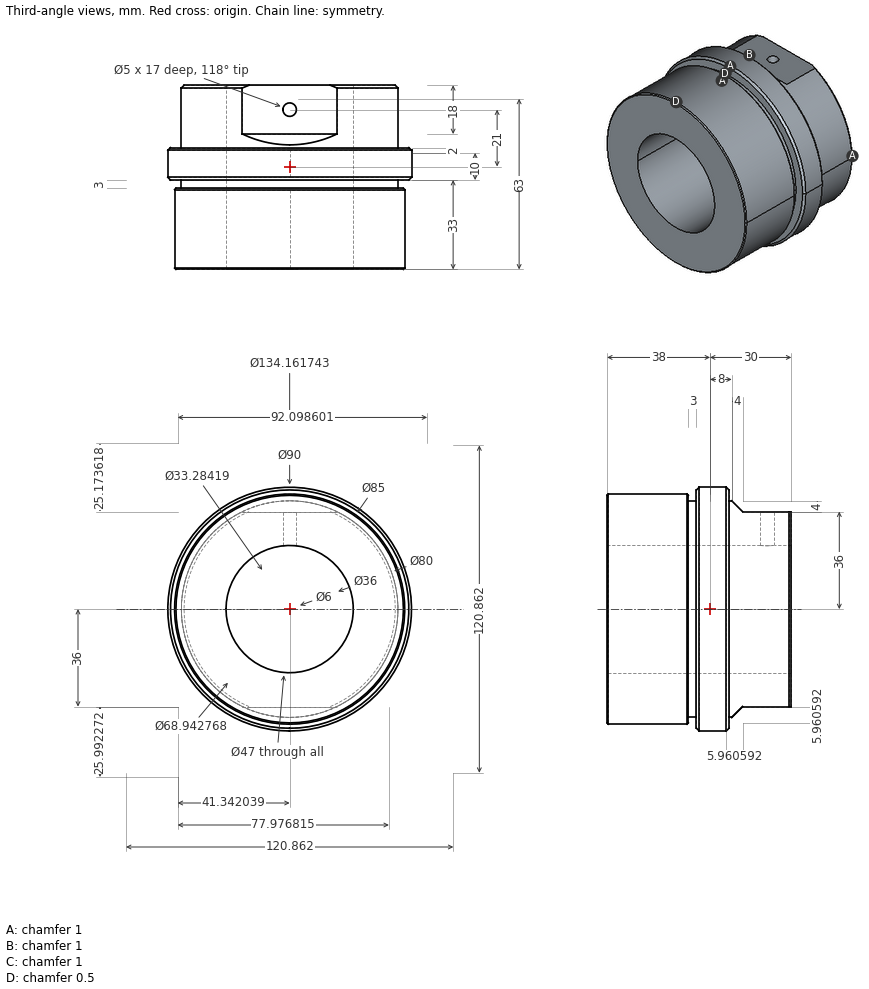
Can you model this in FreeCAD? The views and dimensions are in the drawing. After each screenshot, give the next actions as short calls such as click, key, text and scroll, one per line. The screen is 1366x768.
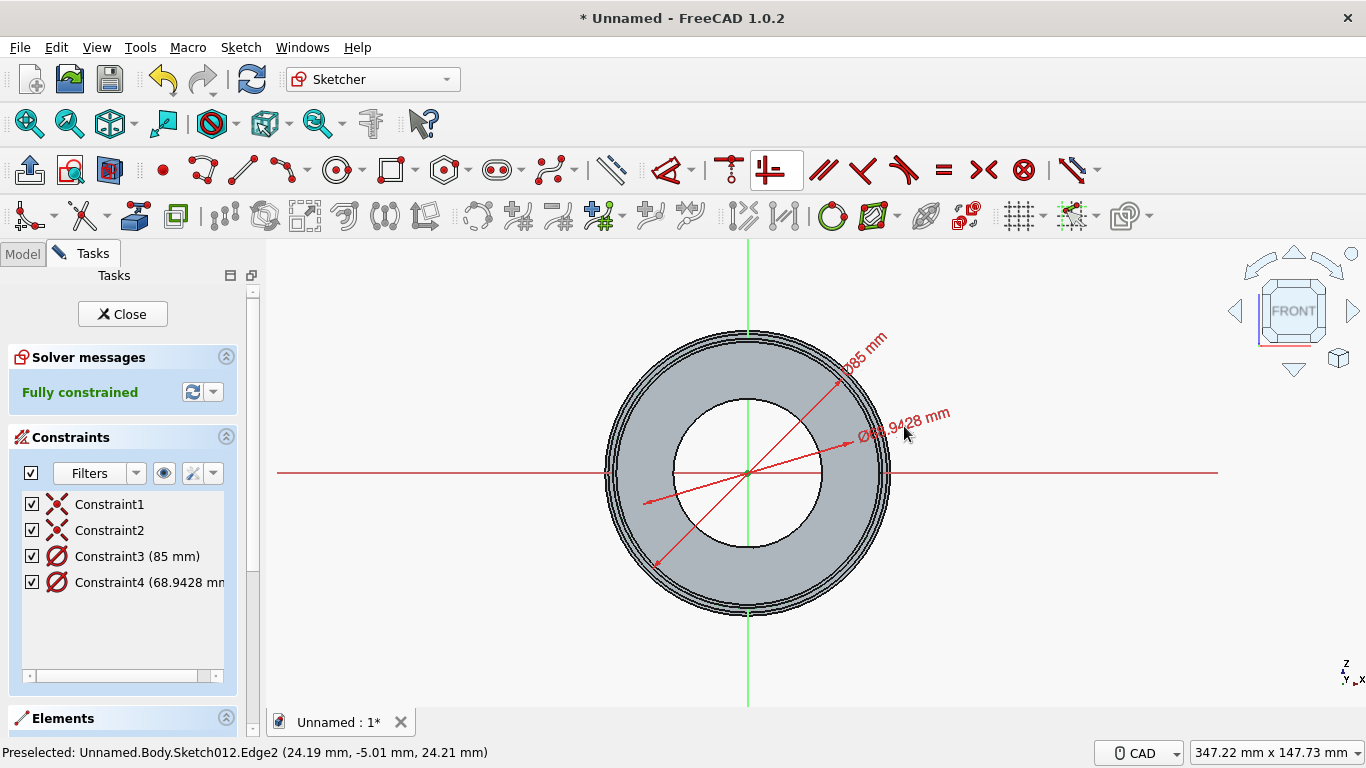
click(123, 314)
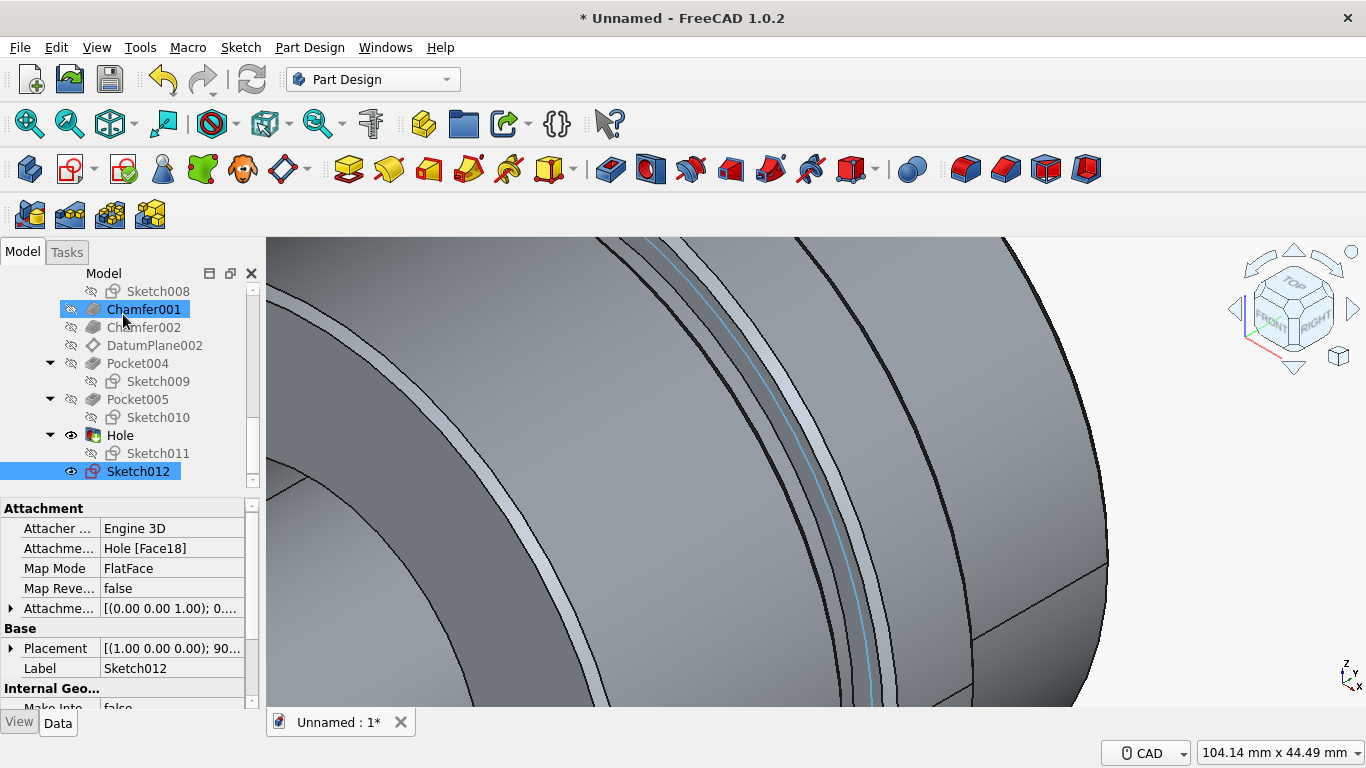
click(350, 170)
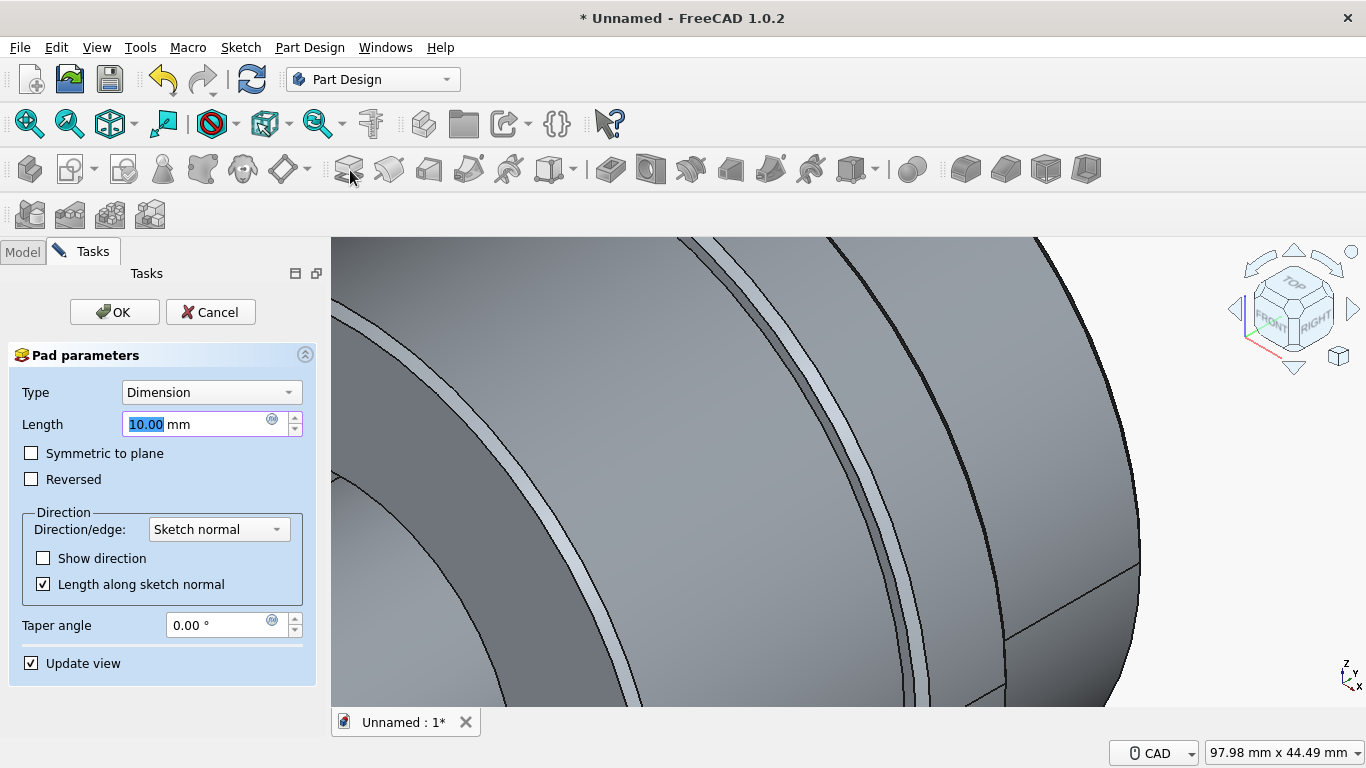
text(33)
key(Tab)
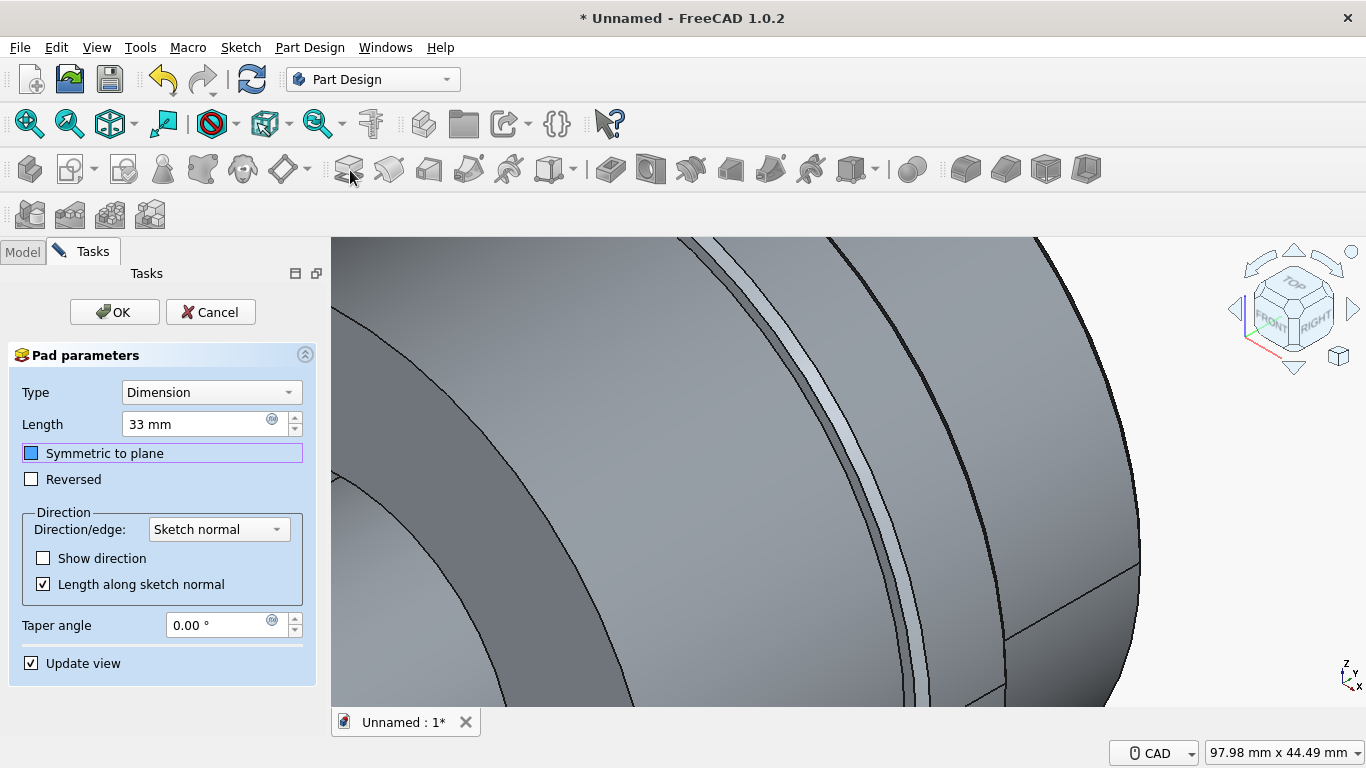
click(115, 312)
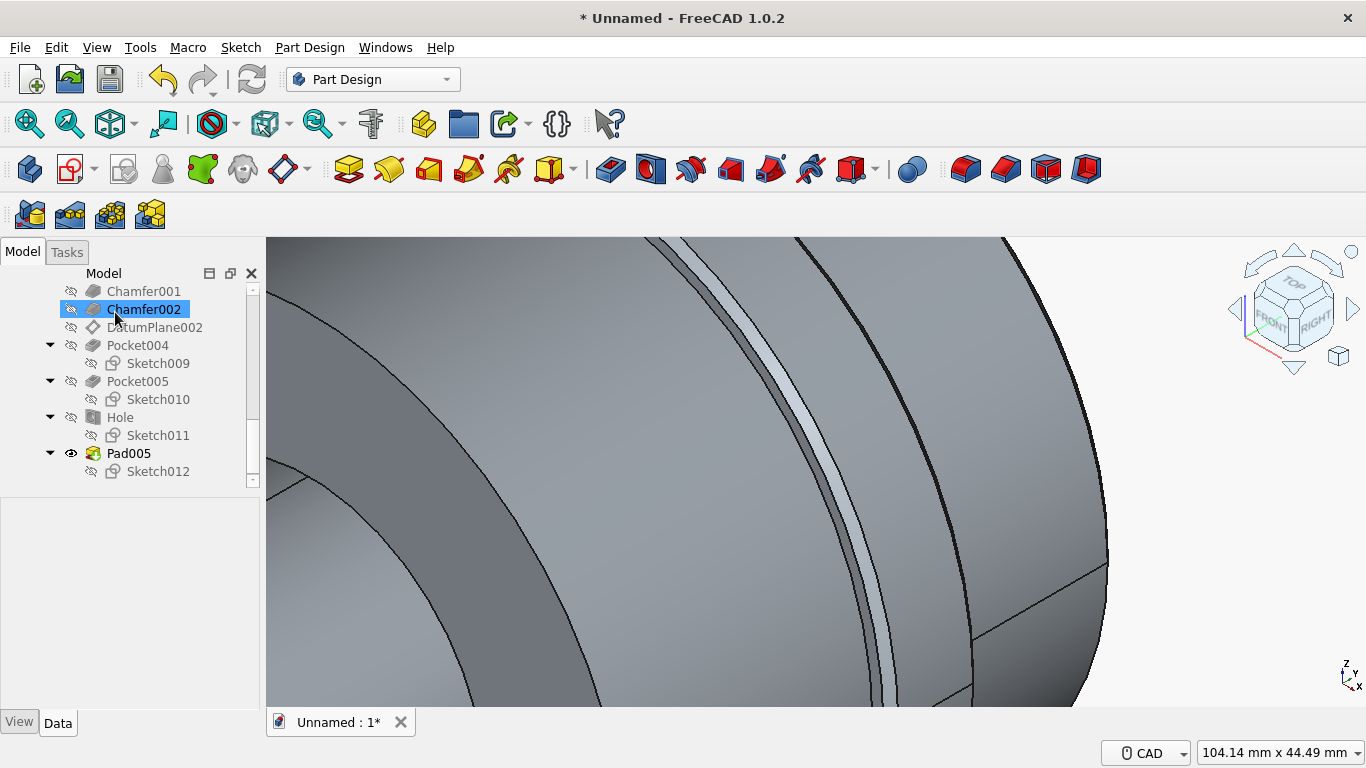
click(30, 124)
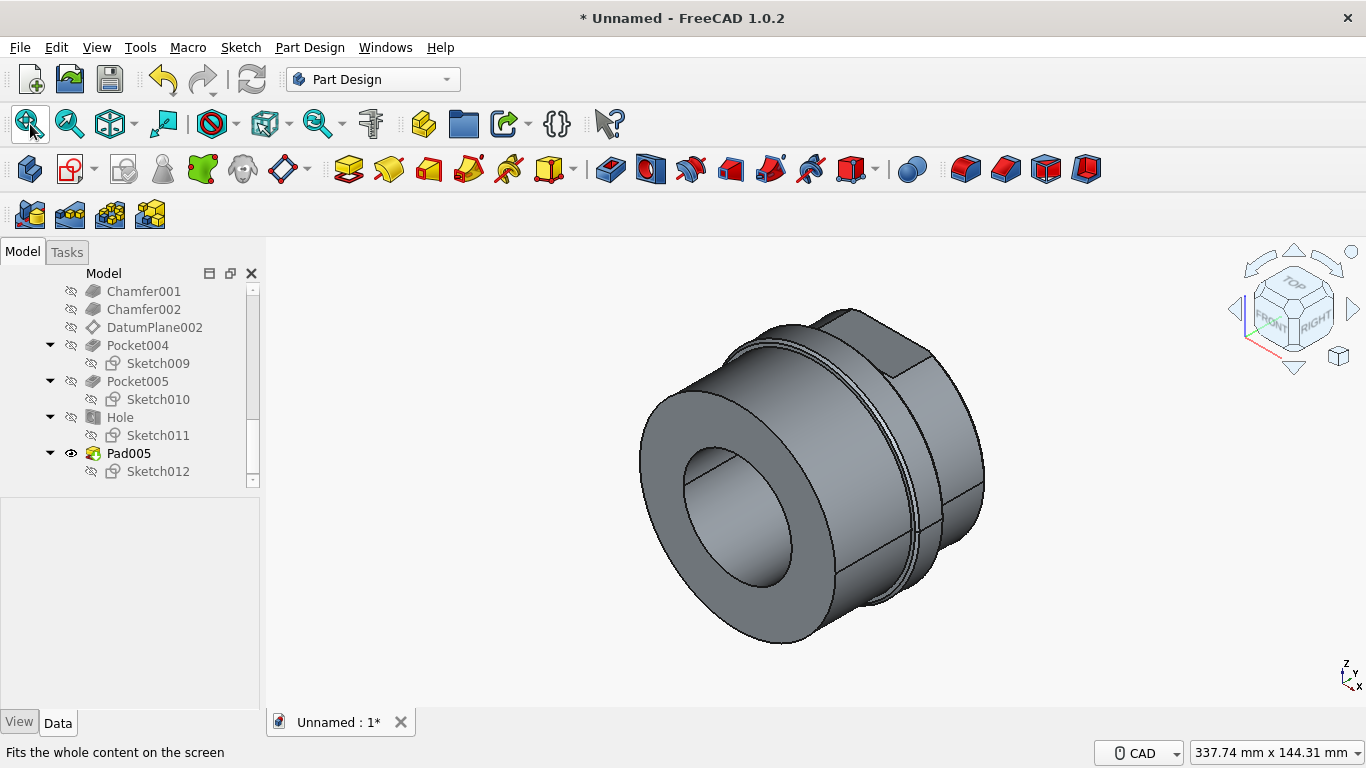
scroll(795, 575, up, 10)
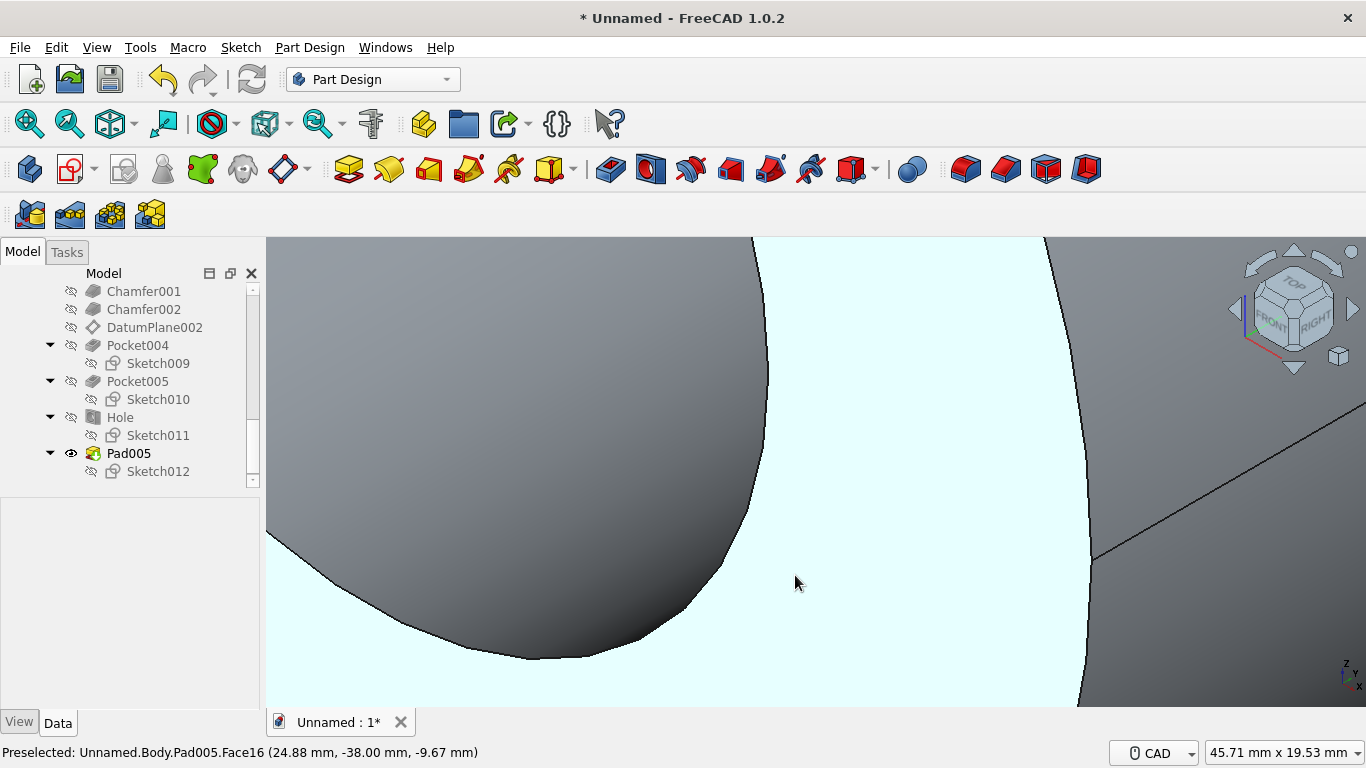
click(30, 124)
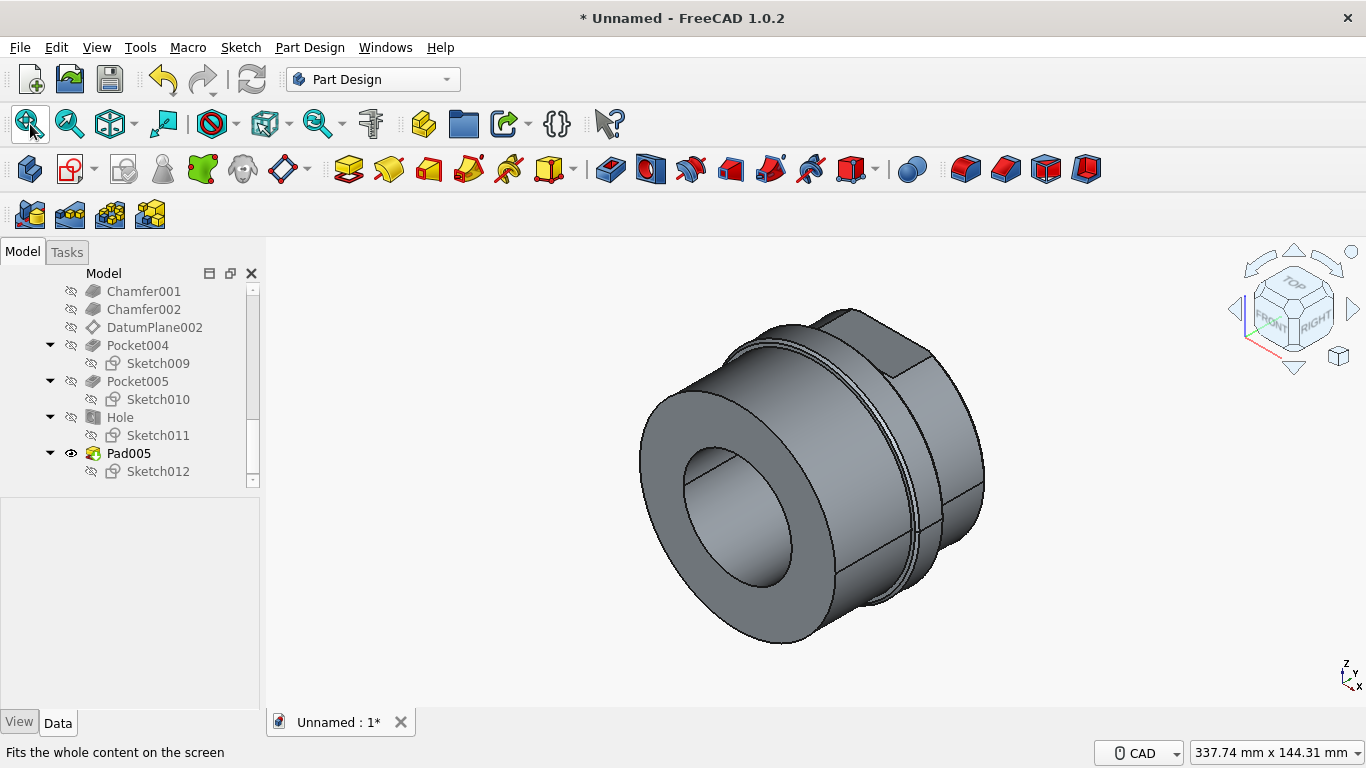
key(1)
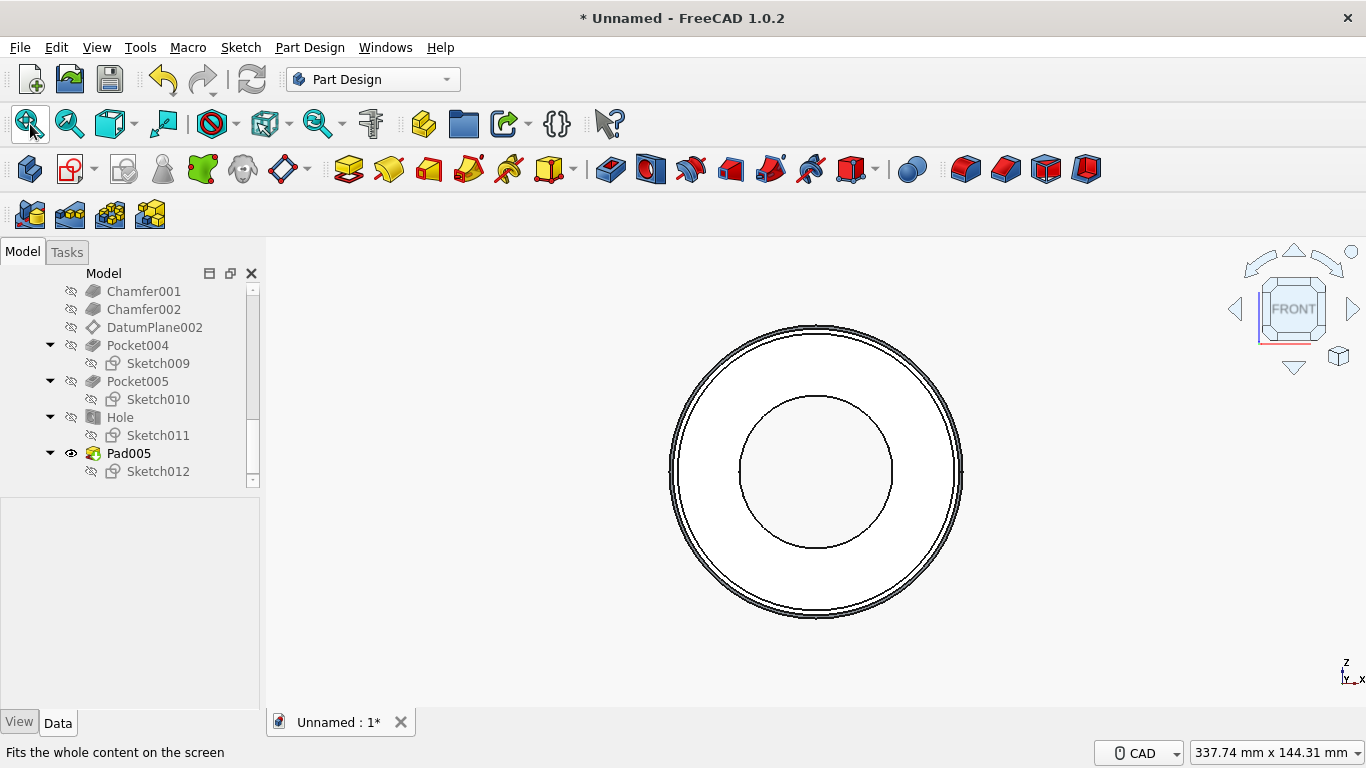
scroll(789, 610, up, 10)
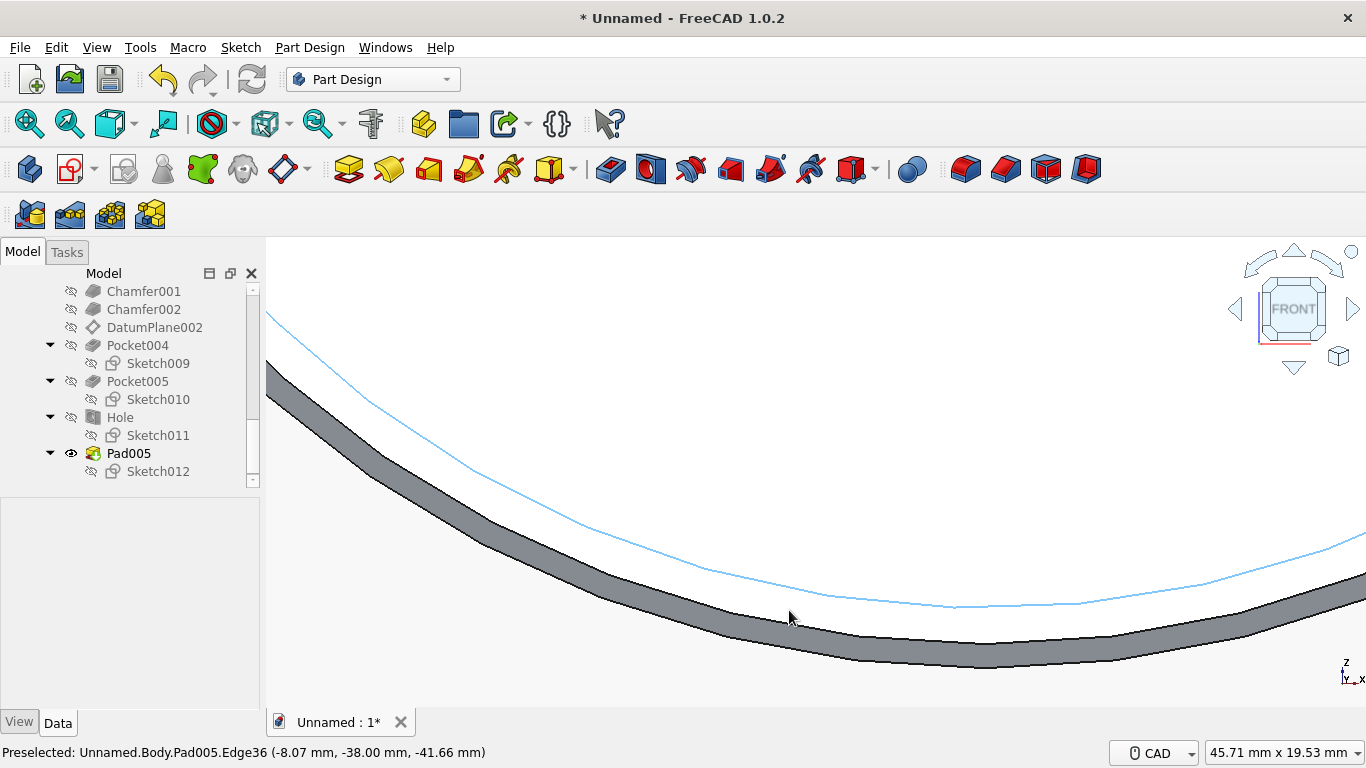
click(786, 612)